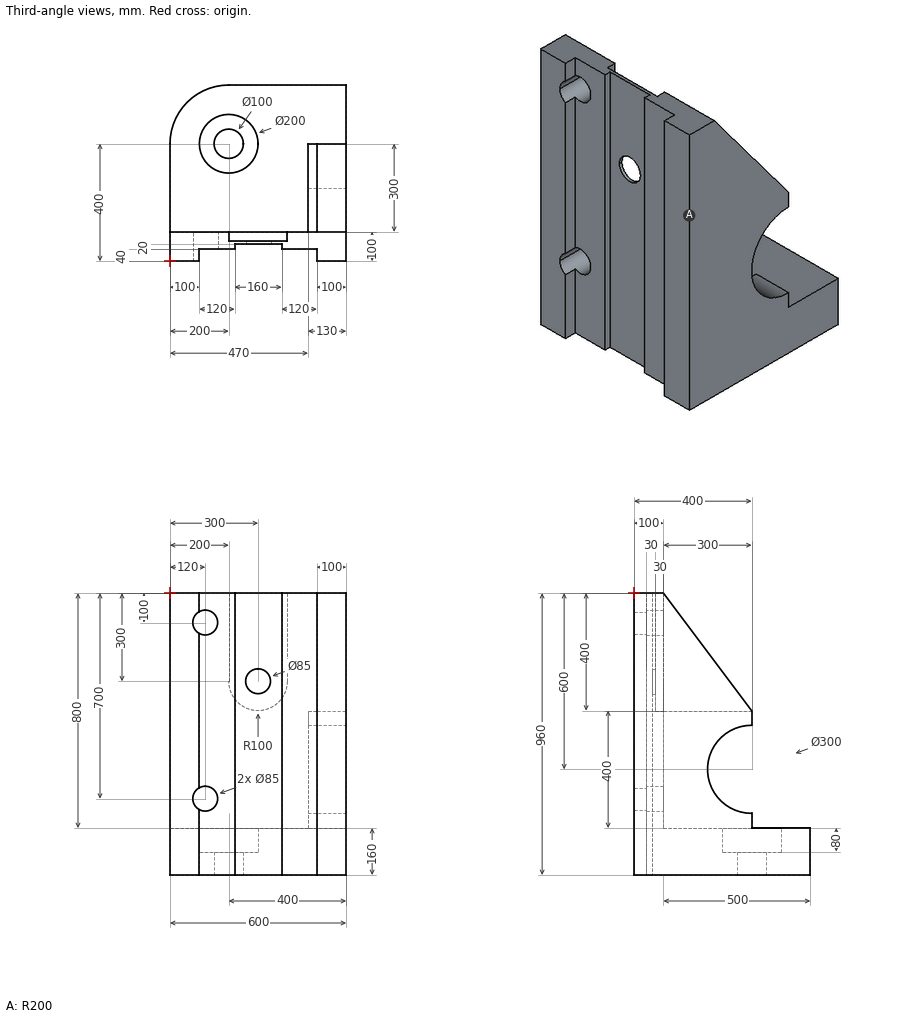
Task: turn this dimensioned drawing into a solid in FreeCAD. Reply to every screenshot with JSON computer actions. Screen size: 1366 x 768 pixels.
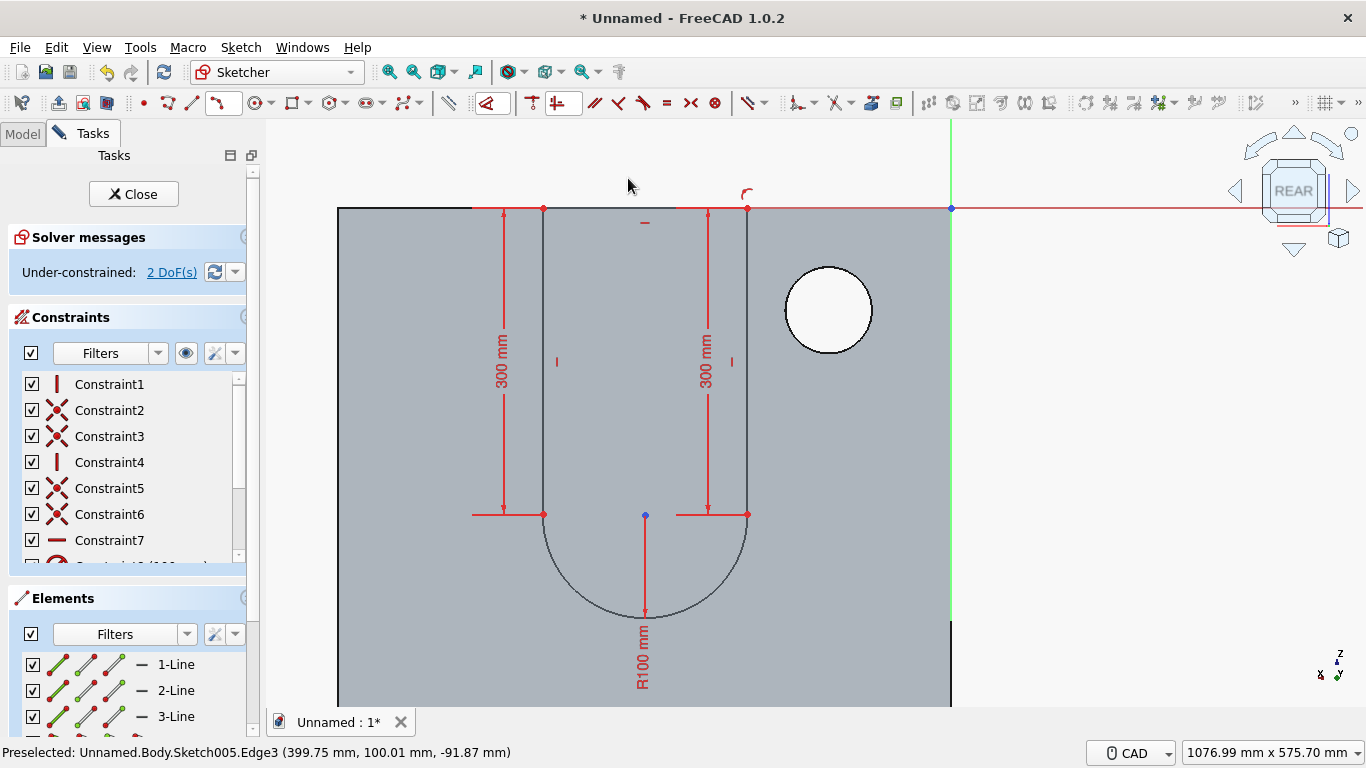
{"action": "left_click", "coordinate": [747, 515]}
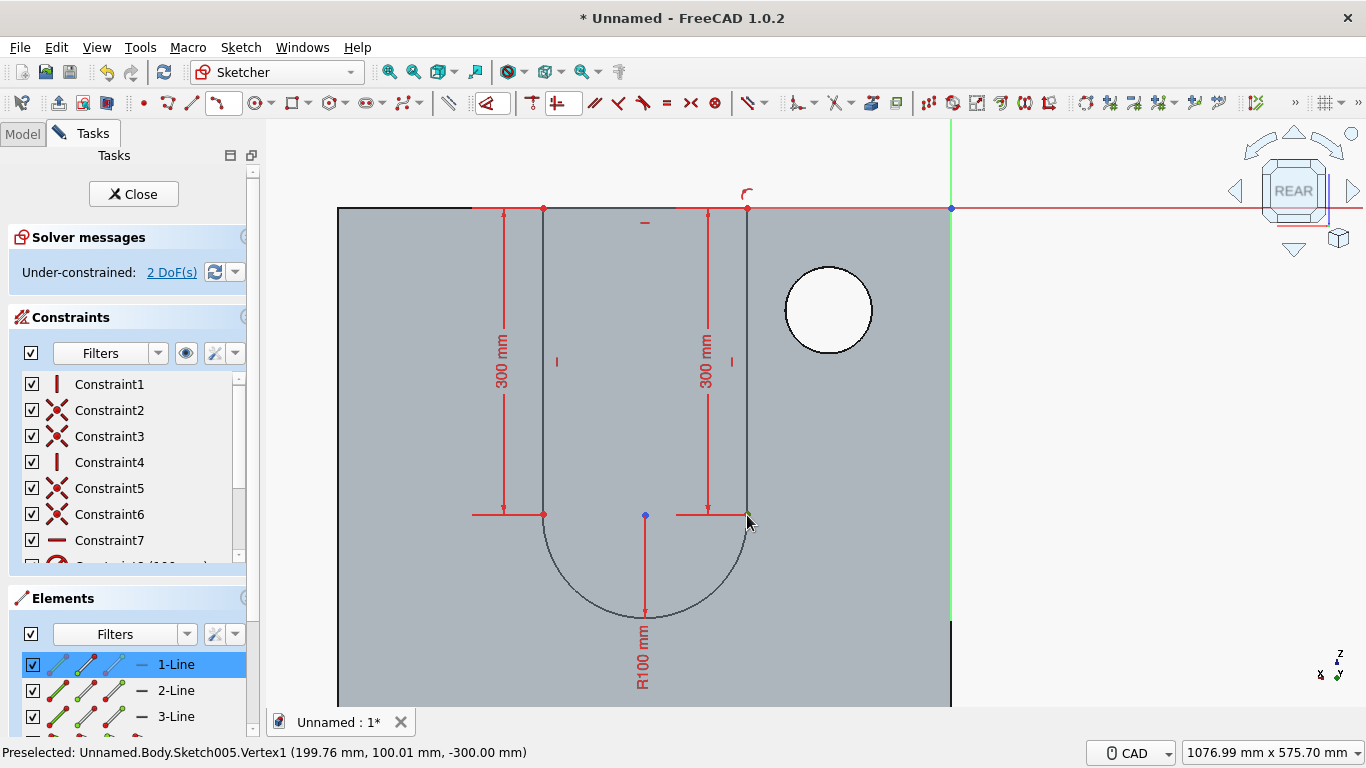
{"action": "left_click", "coordinate": [504, 104]}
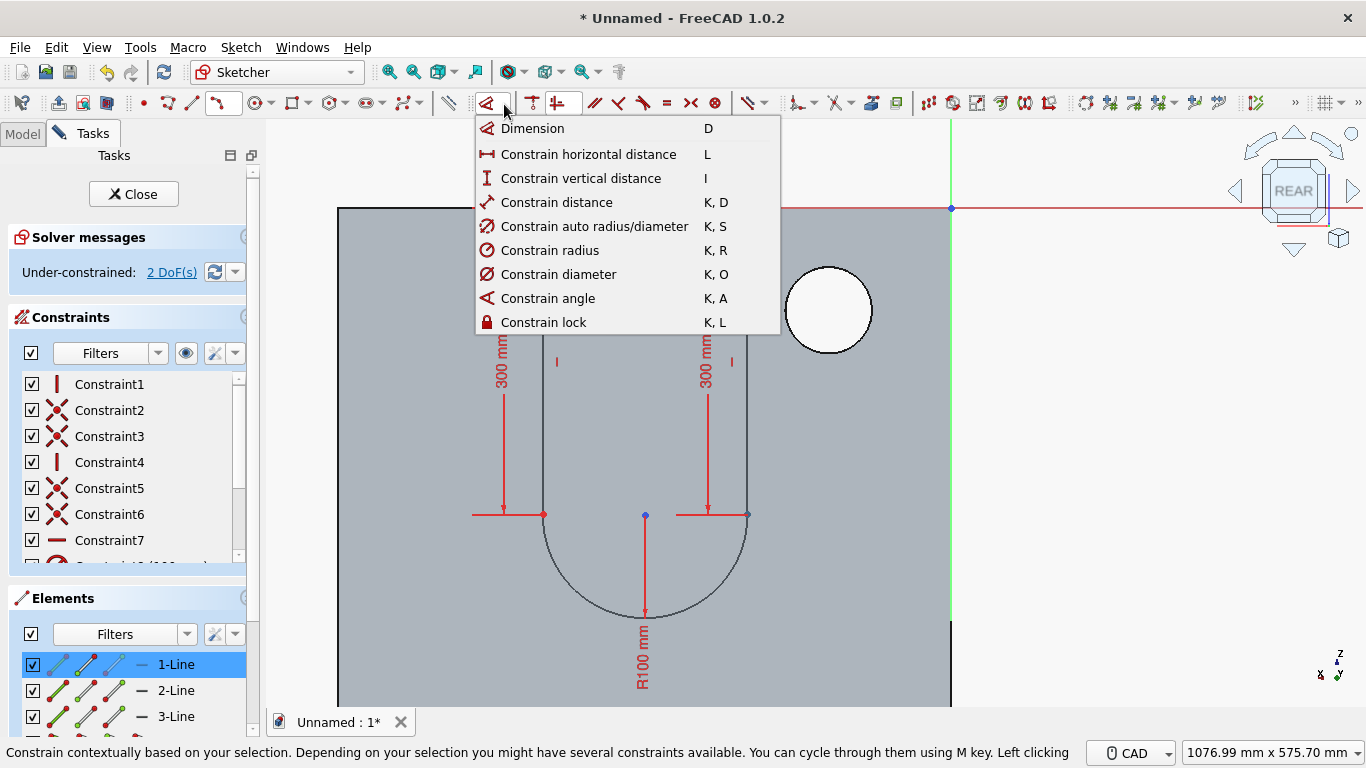
{"action": "left_click", "coordinate": [628, 154]}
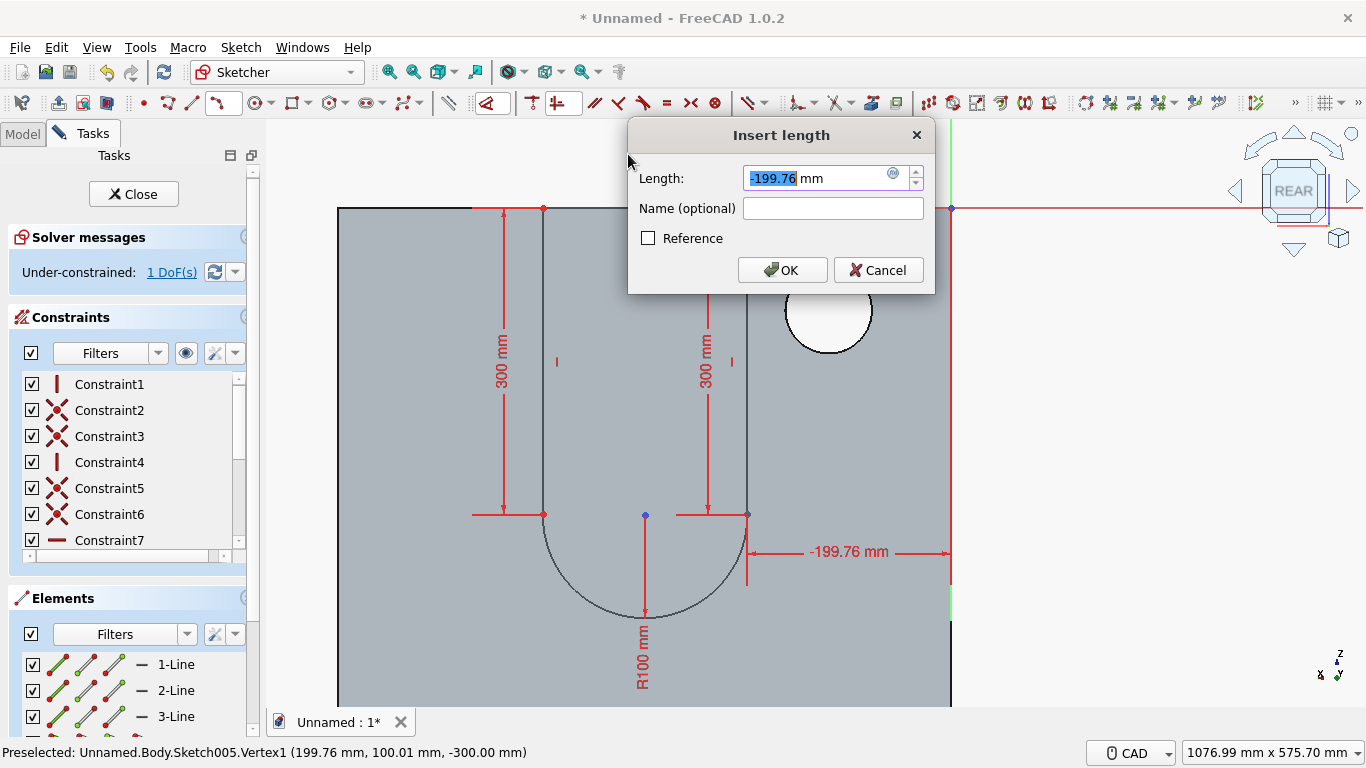
{"action": "type", "text": "-200"}
{"action": "key", "text": "Return"}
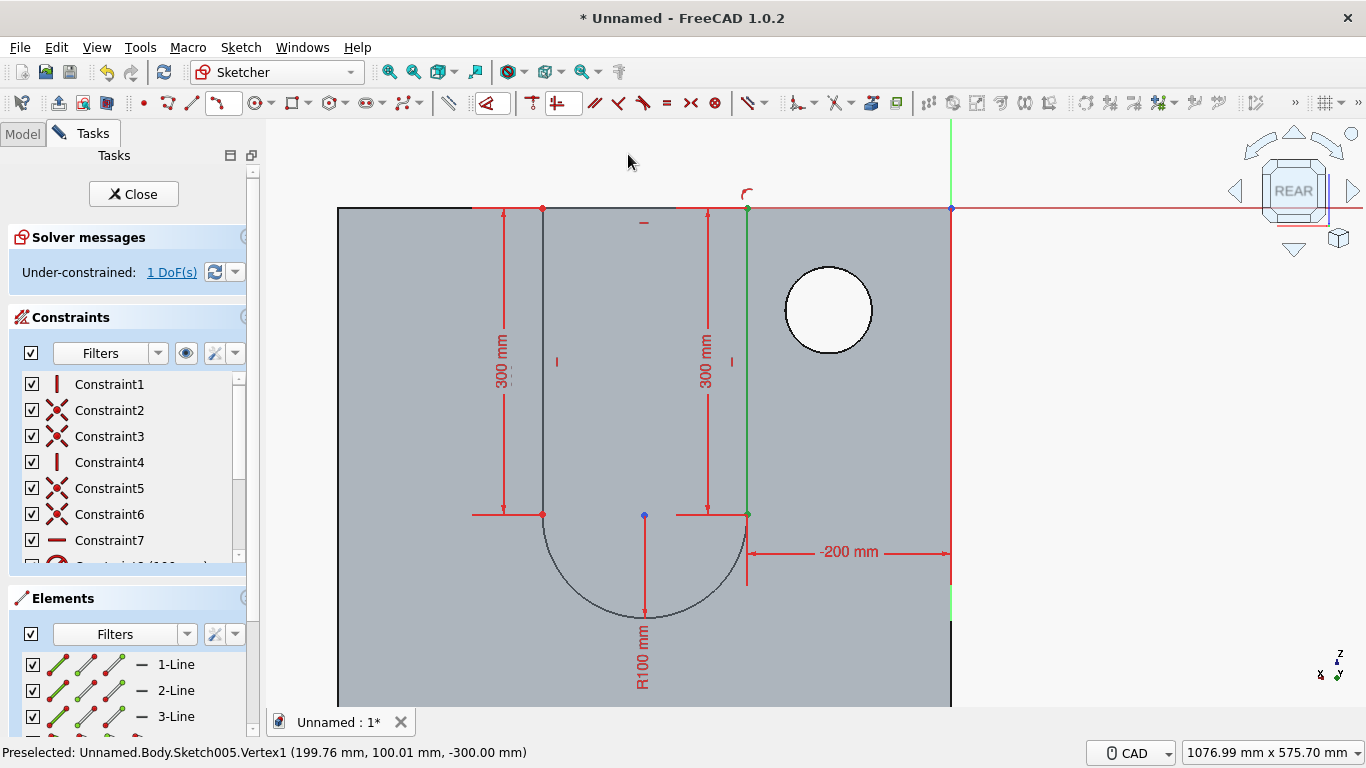
{"action": "left_click", "coordinate": [645, 516]}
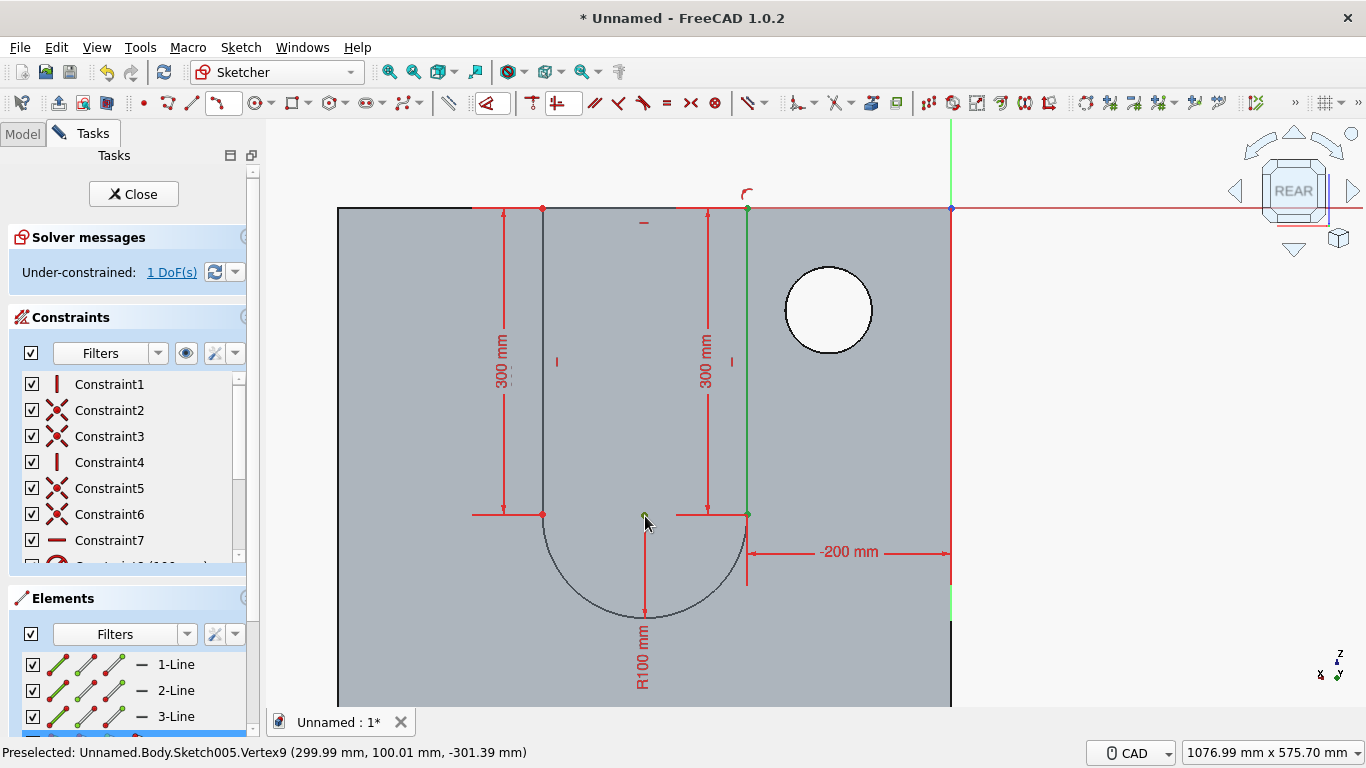
{"action": "key", "text": "i"}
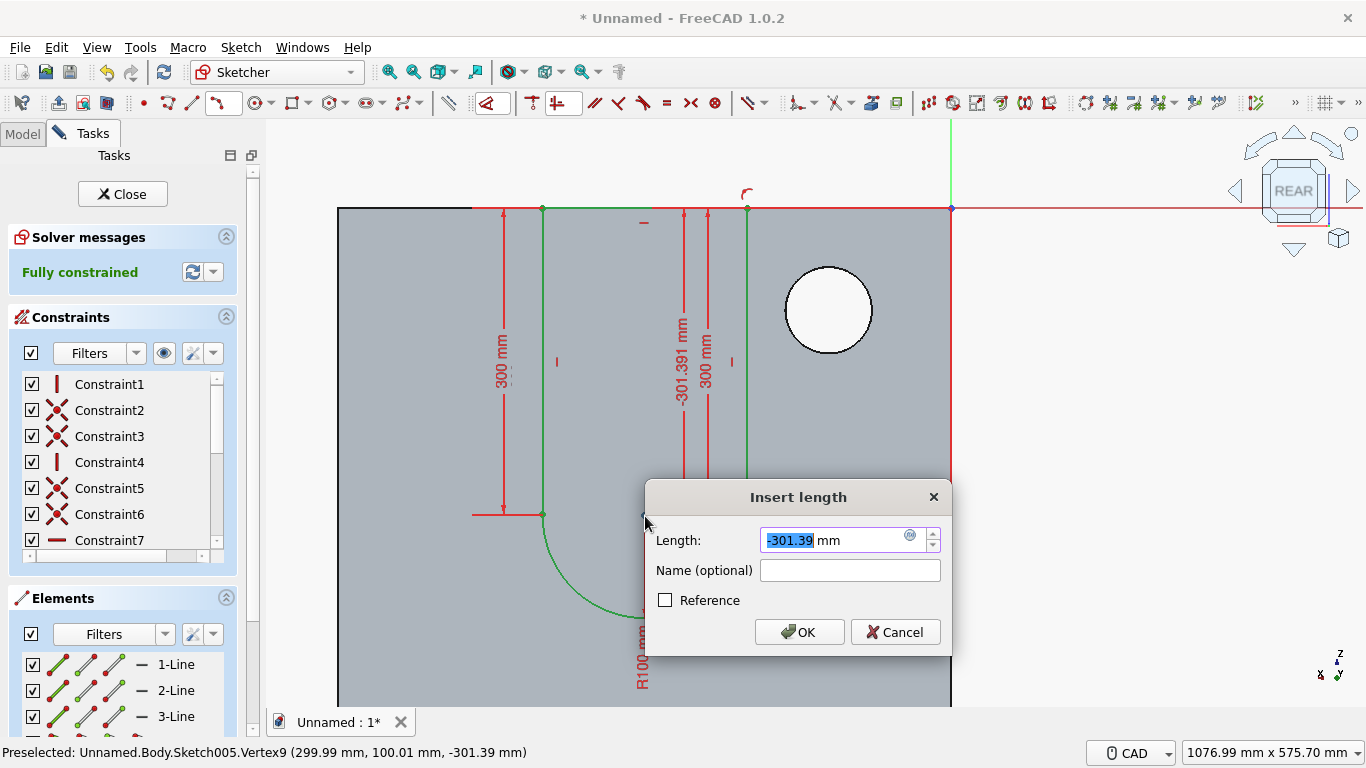
{"action": "type", "text": "-300"}
{"action": "key", "text": "Return"}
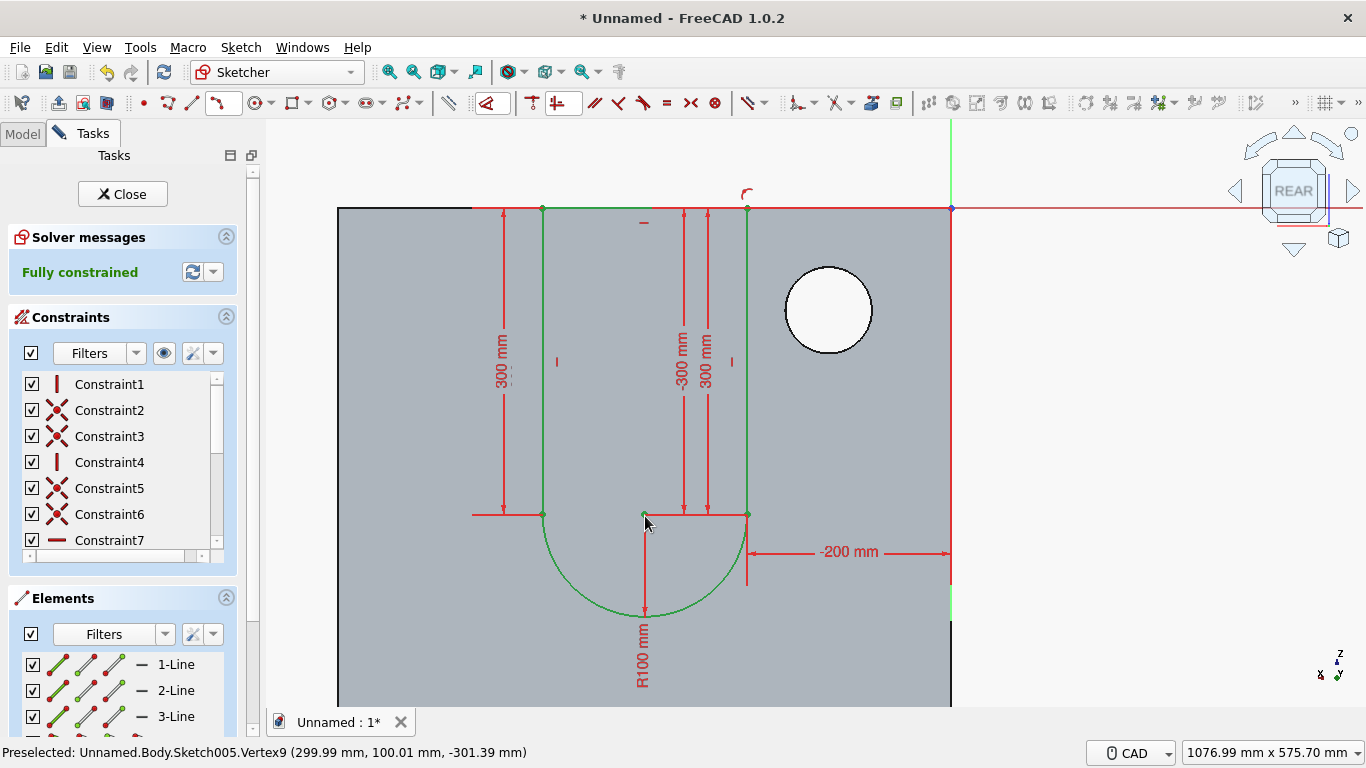
{"action": "left_click", "coordinate": [123, 194]}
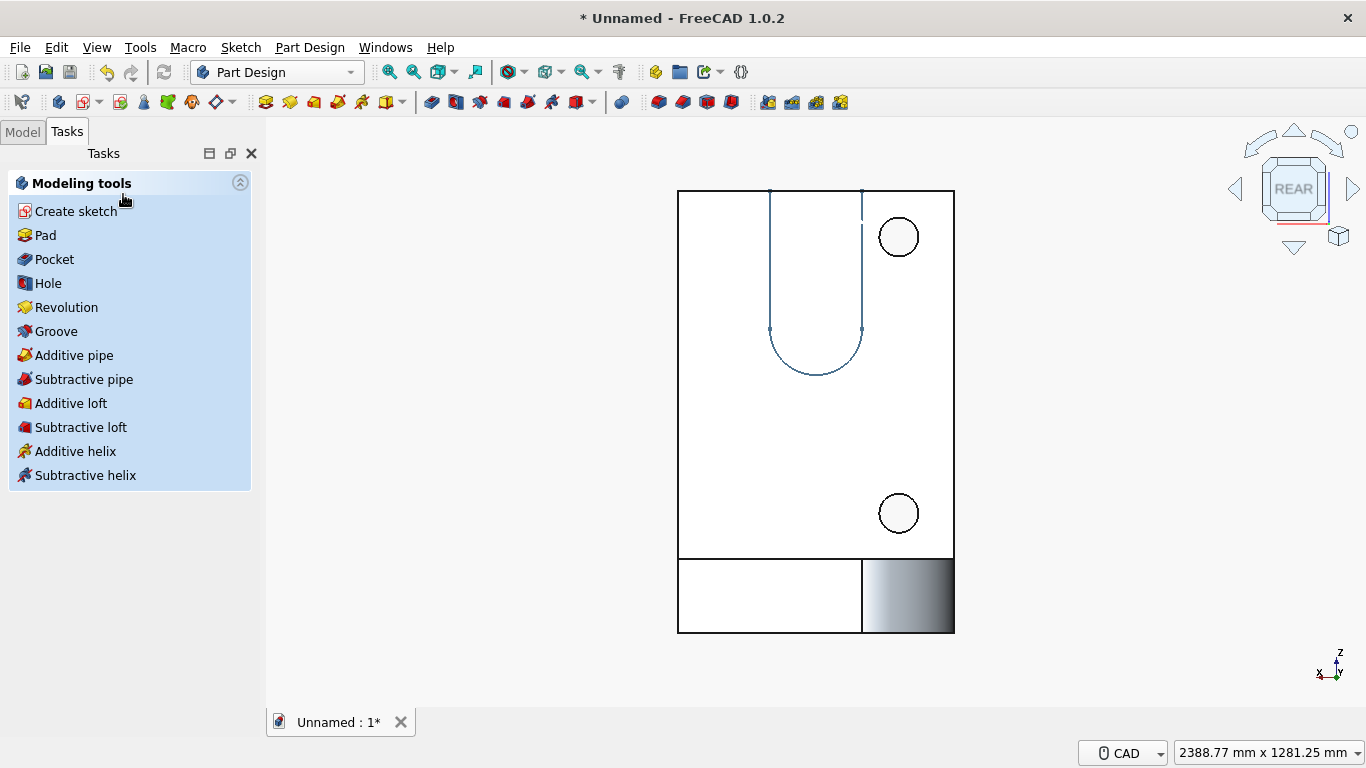
{"action": "left_click", "coordinate": [432, 102]}